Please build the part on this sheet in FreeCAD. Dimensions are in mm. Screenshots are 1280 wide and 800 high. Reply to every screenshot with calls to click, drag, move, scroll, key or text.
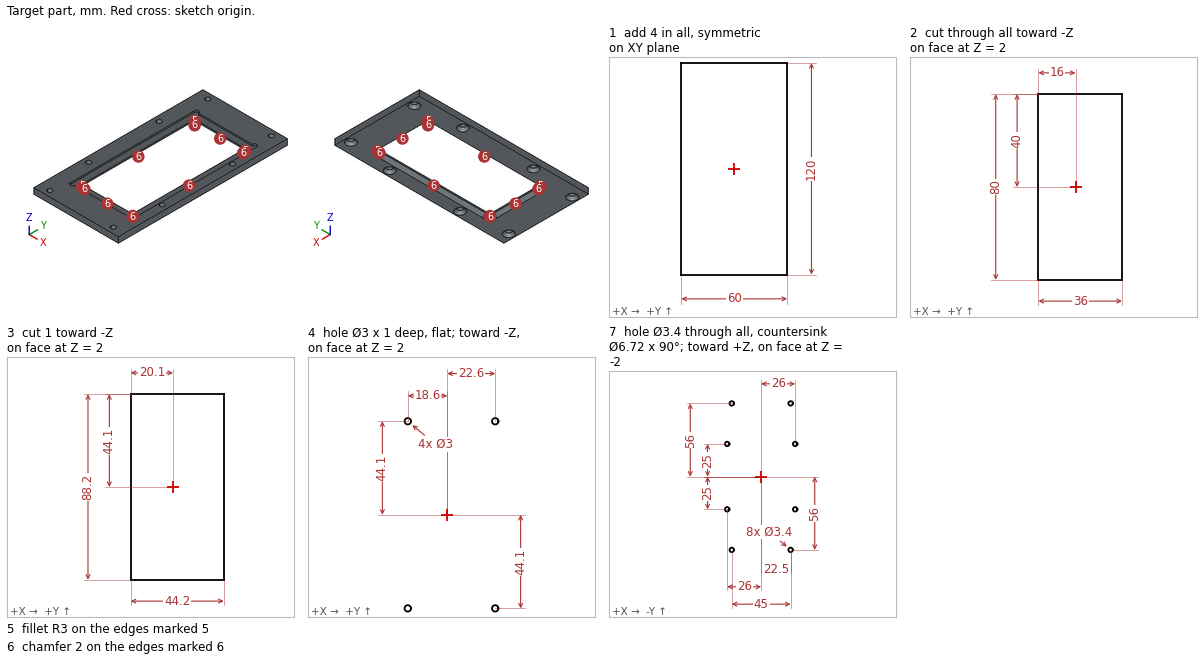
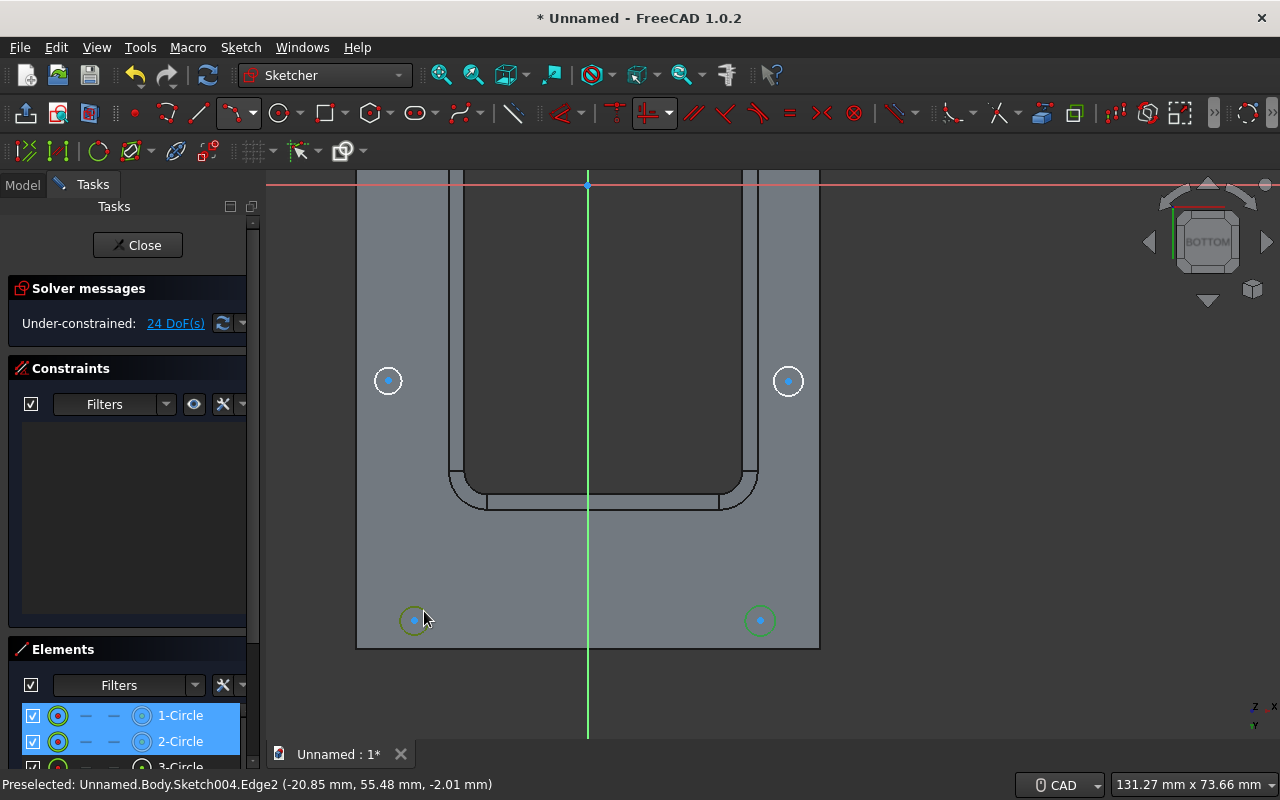
click(398, 372)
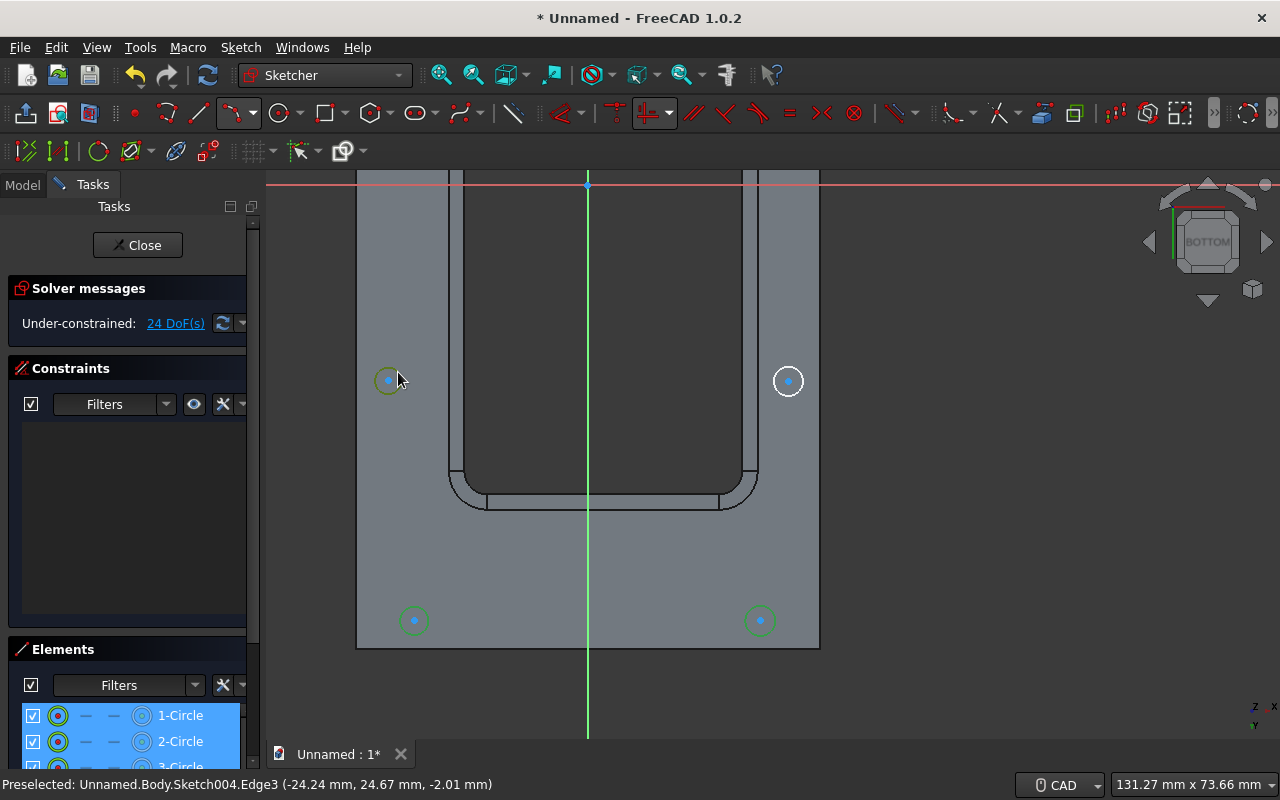
scroll(772, 611, down, 5)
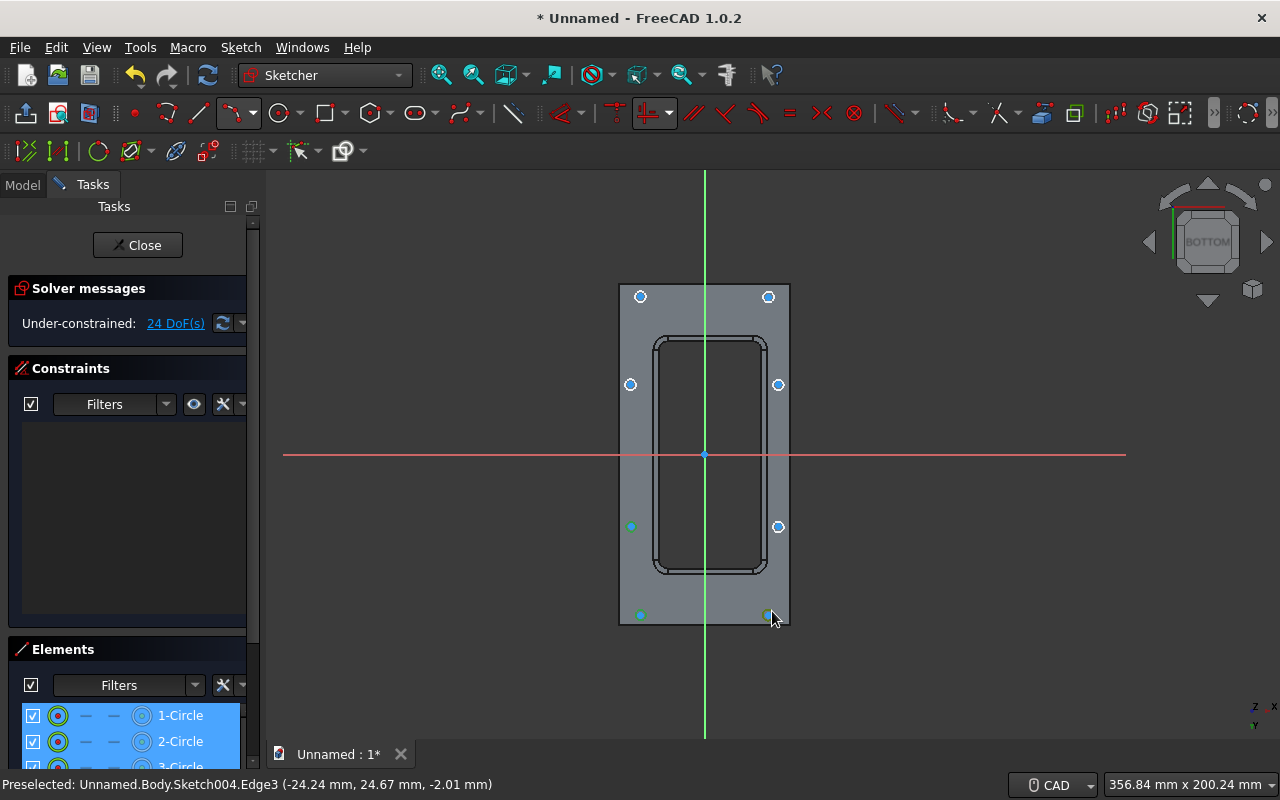
scroll(634, 381, up, 5)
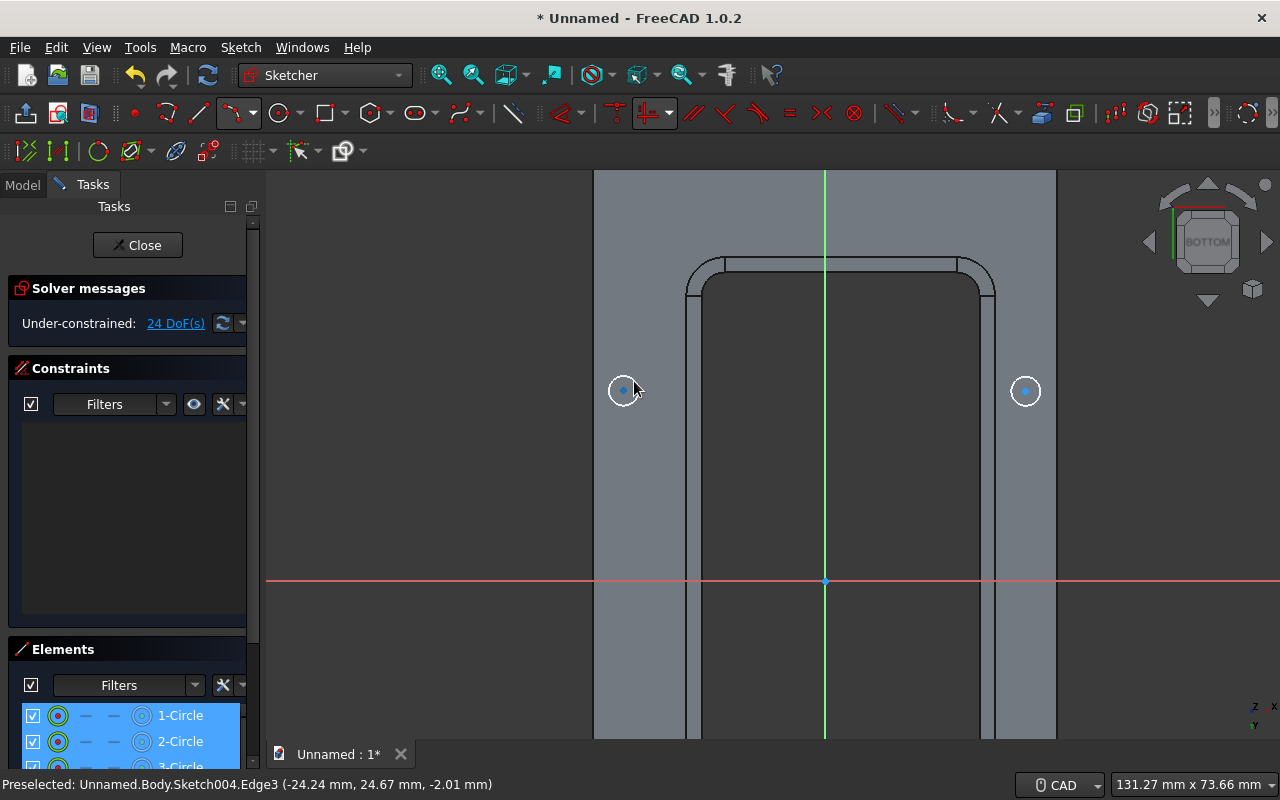
click(634, 380)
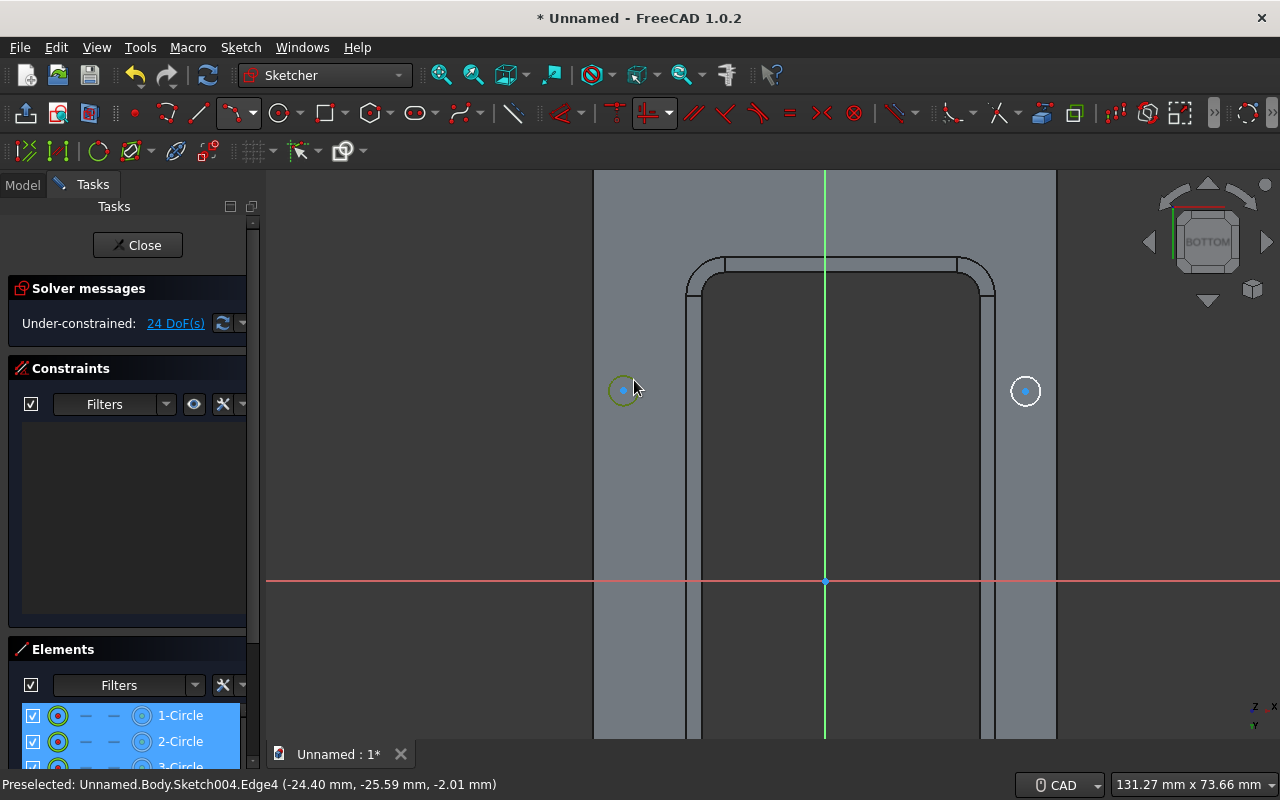
scroll(634, 381, down, 5)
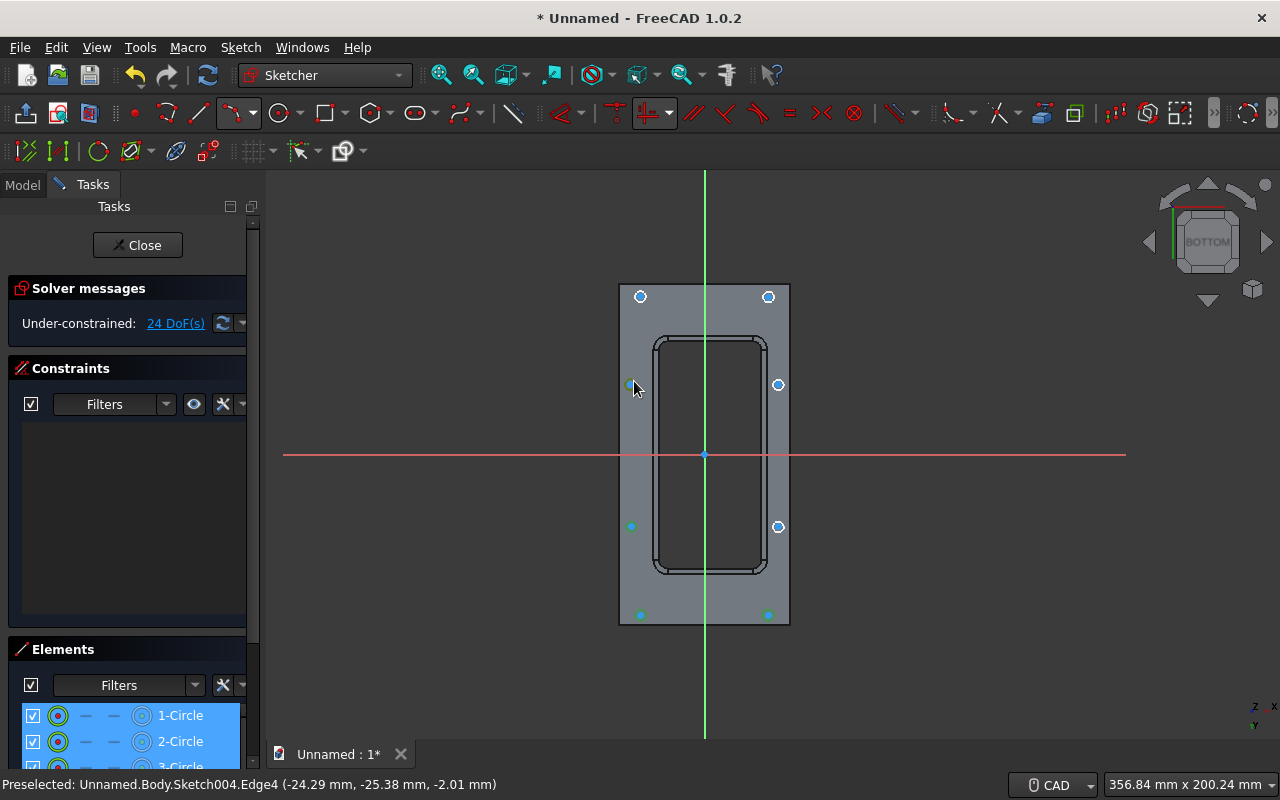
scroll(644, 293, up, 5)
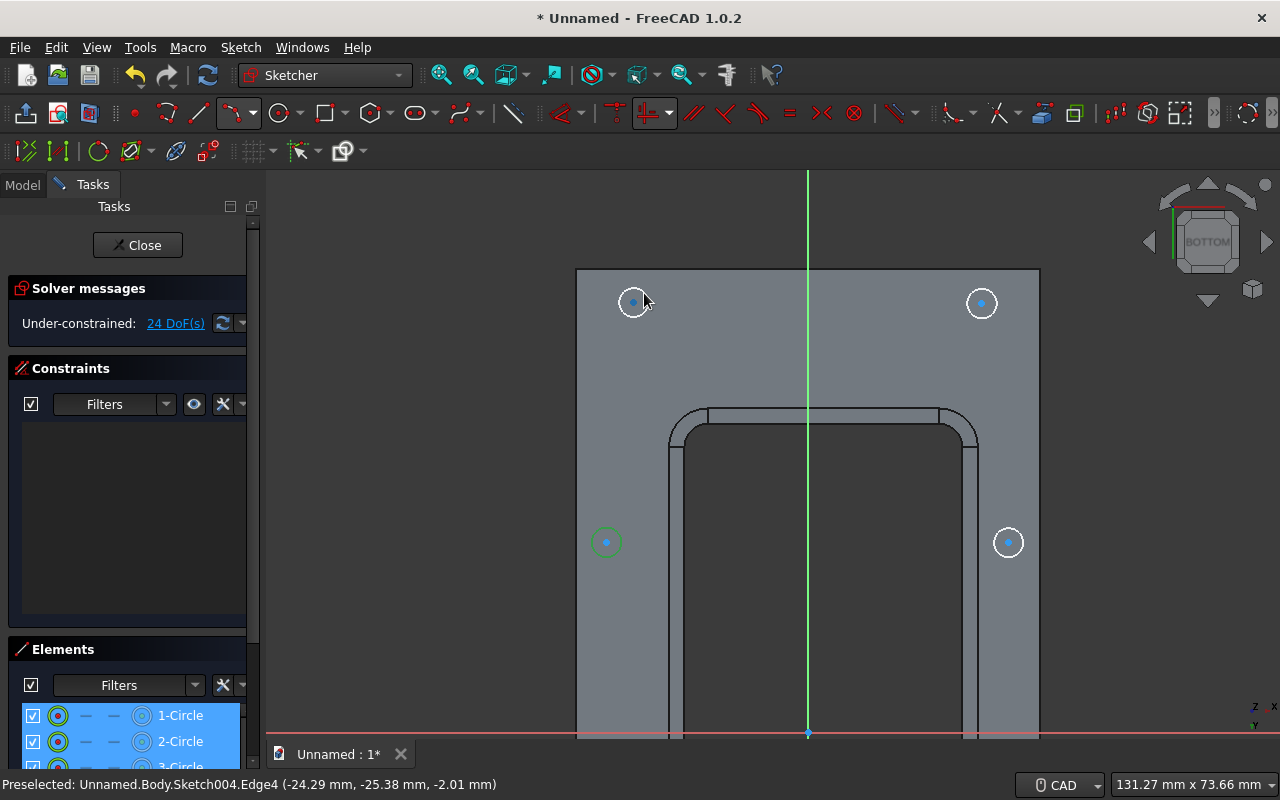
click(644, 292)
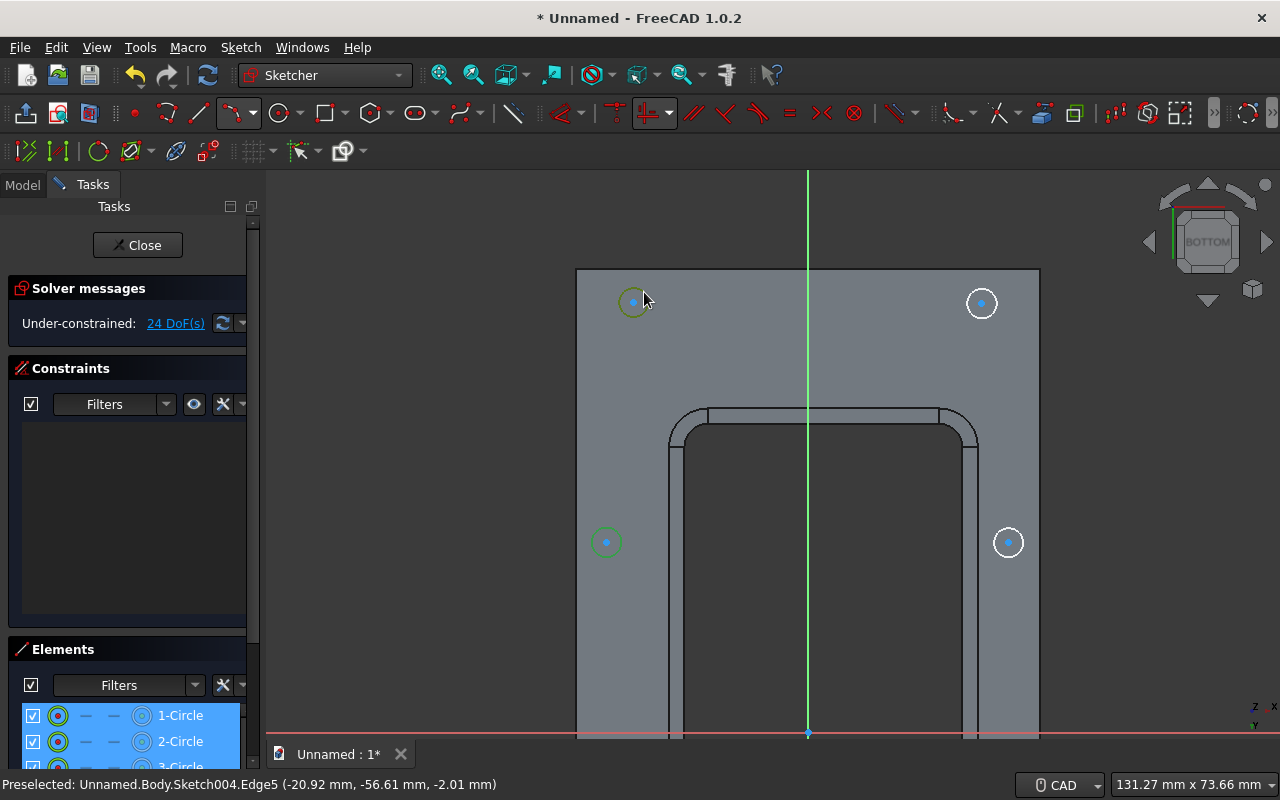
click(992, 293)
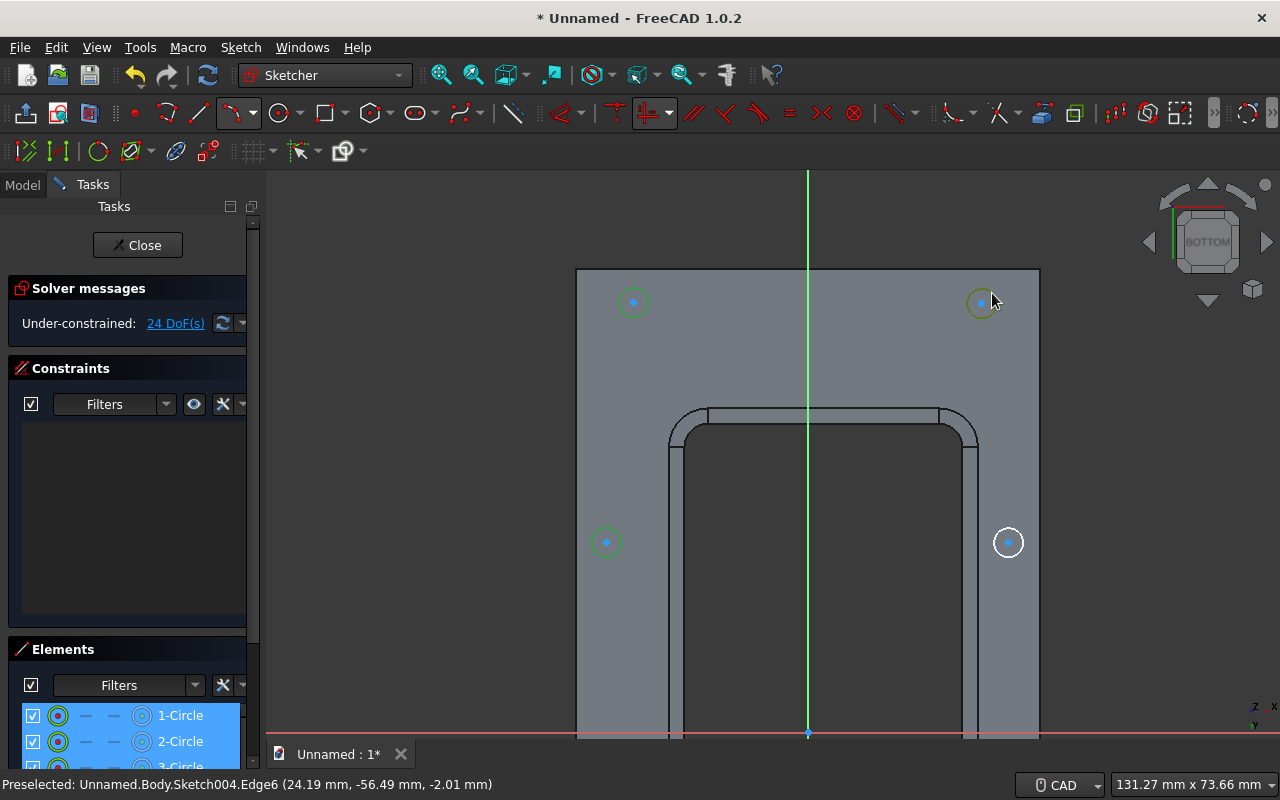
click(1019, 532)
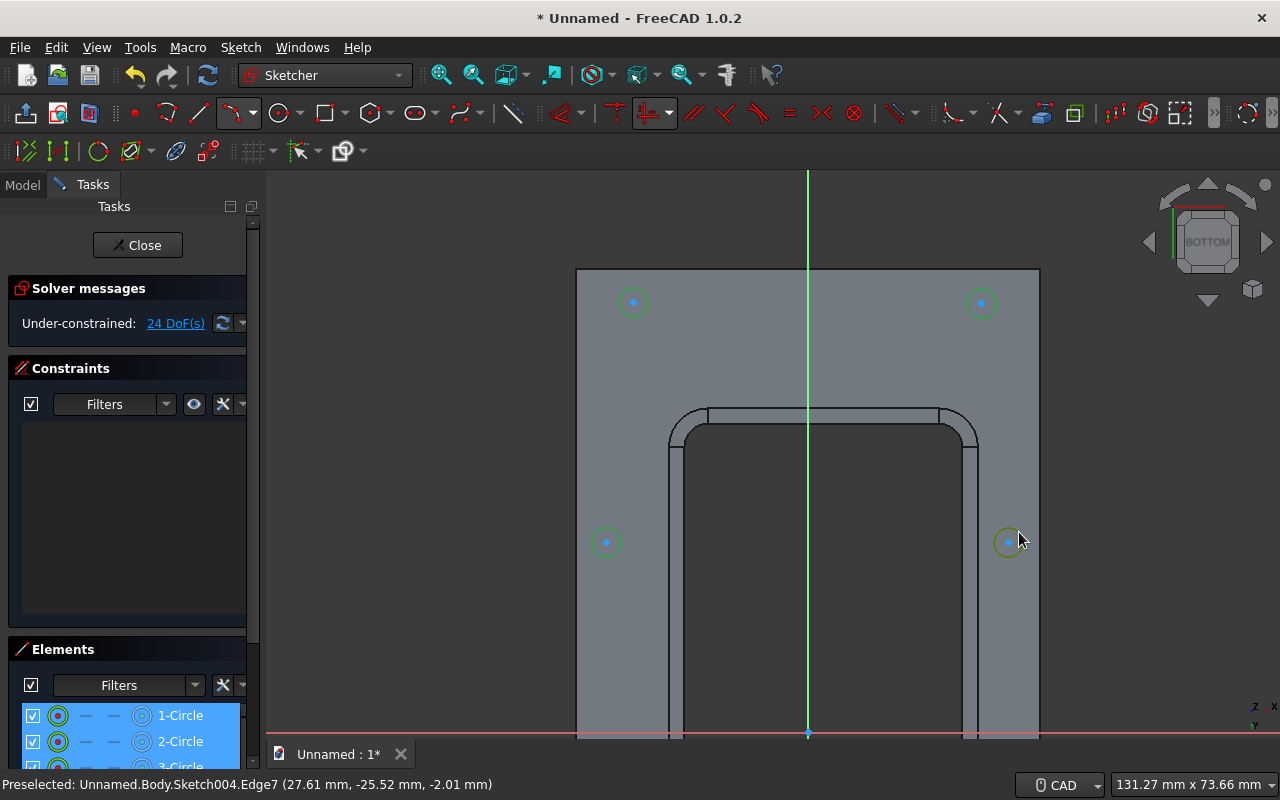
scroll(644, 293, down, 5)